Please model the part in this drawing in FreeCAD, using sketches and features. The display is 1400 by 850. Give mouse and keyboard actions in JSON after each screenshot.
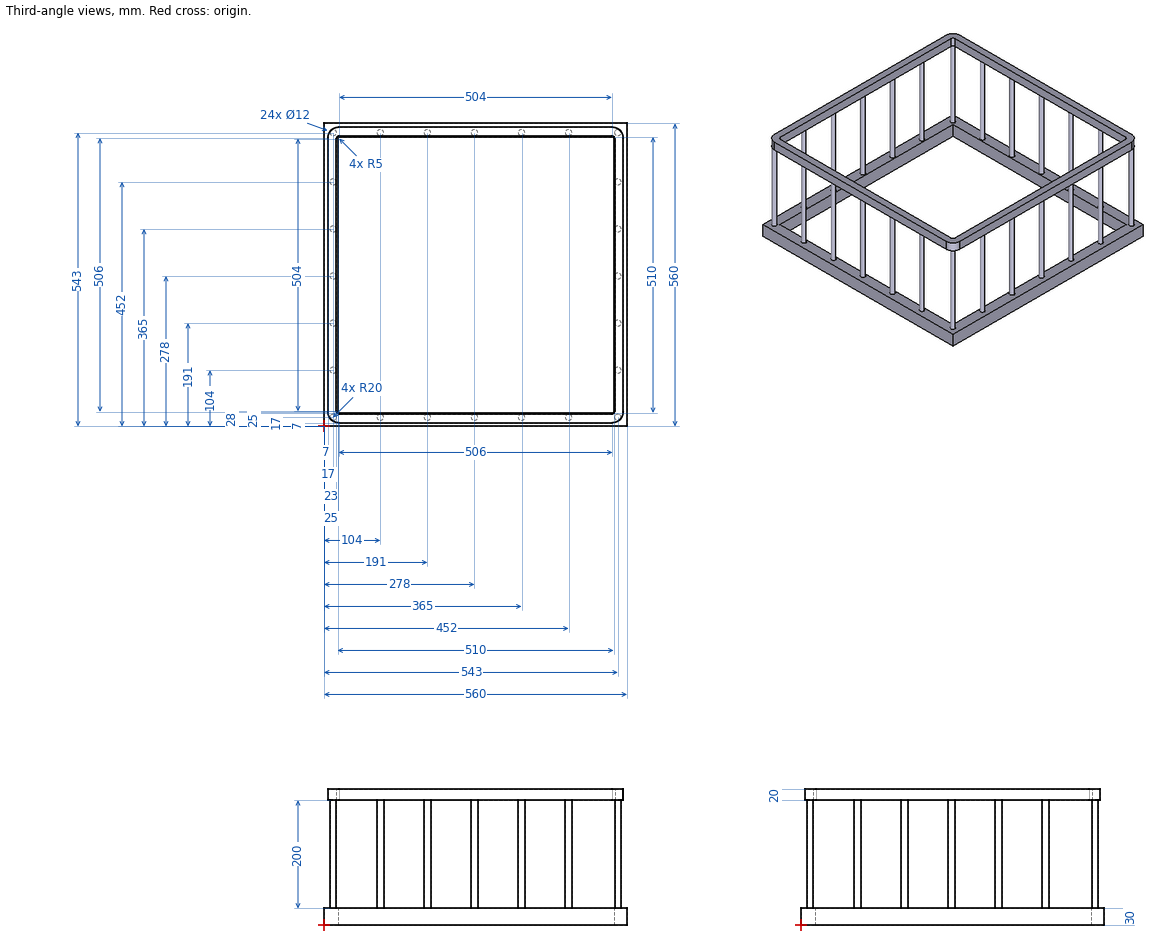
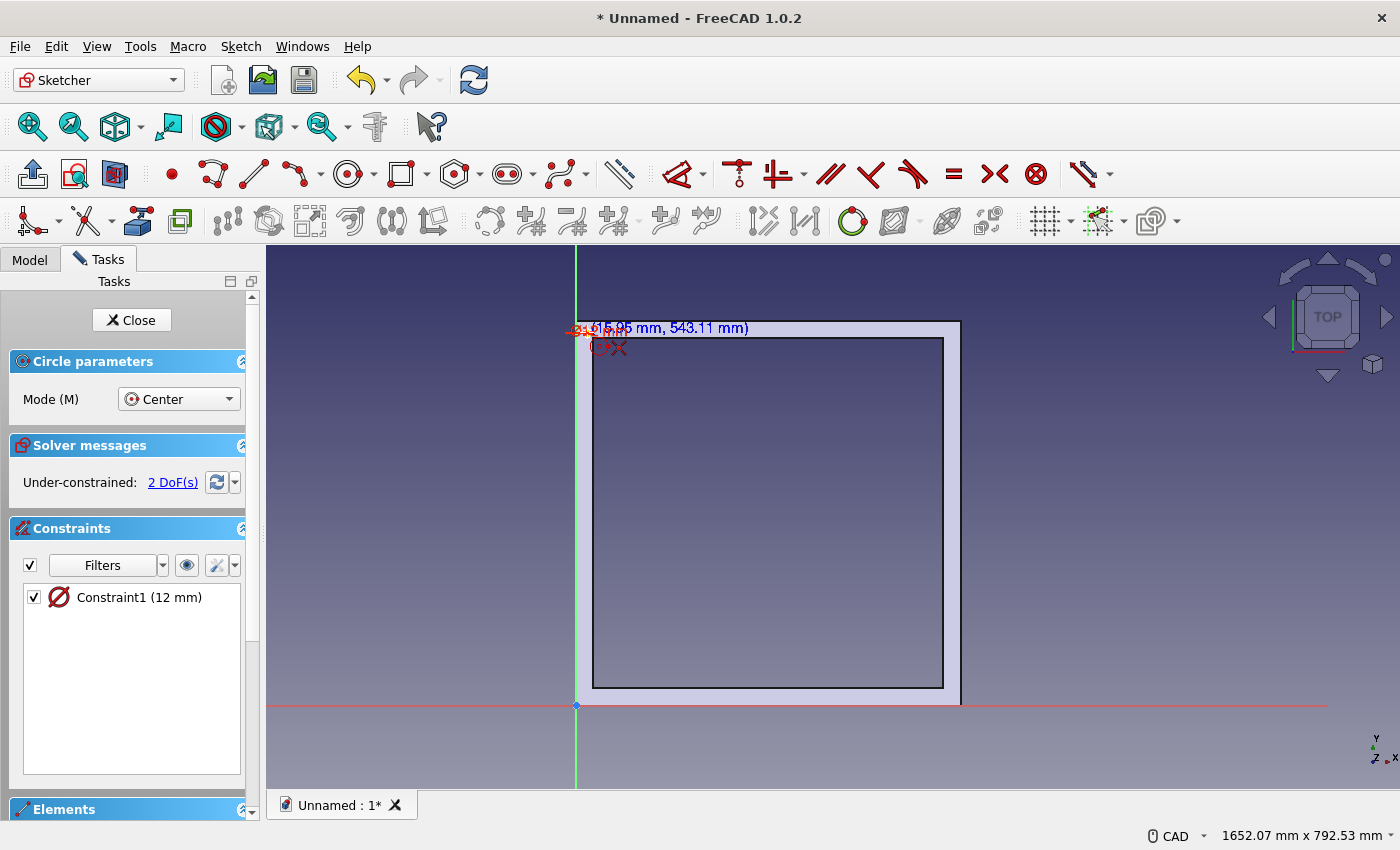
{"action": "scroll", "coordinate": [588, 694], "scroll_direction": "up", "scroll_amount": 9}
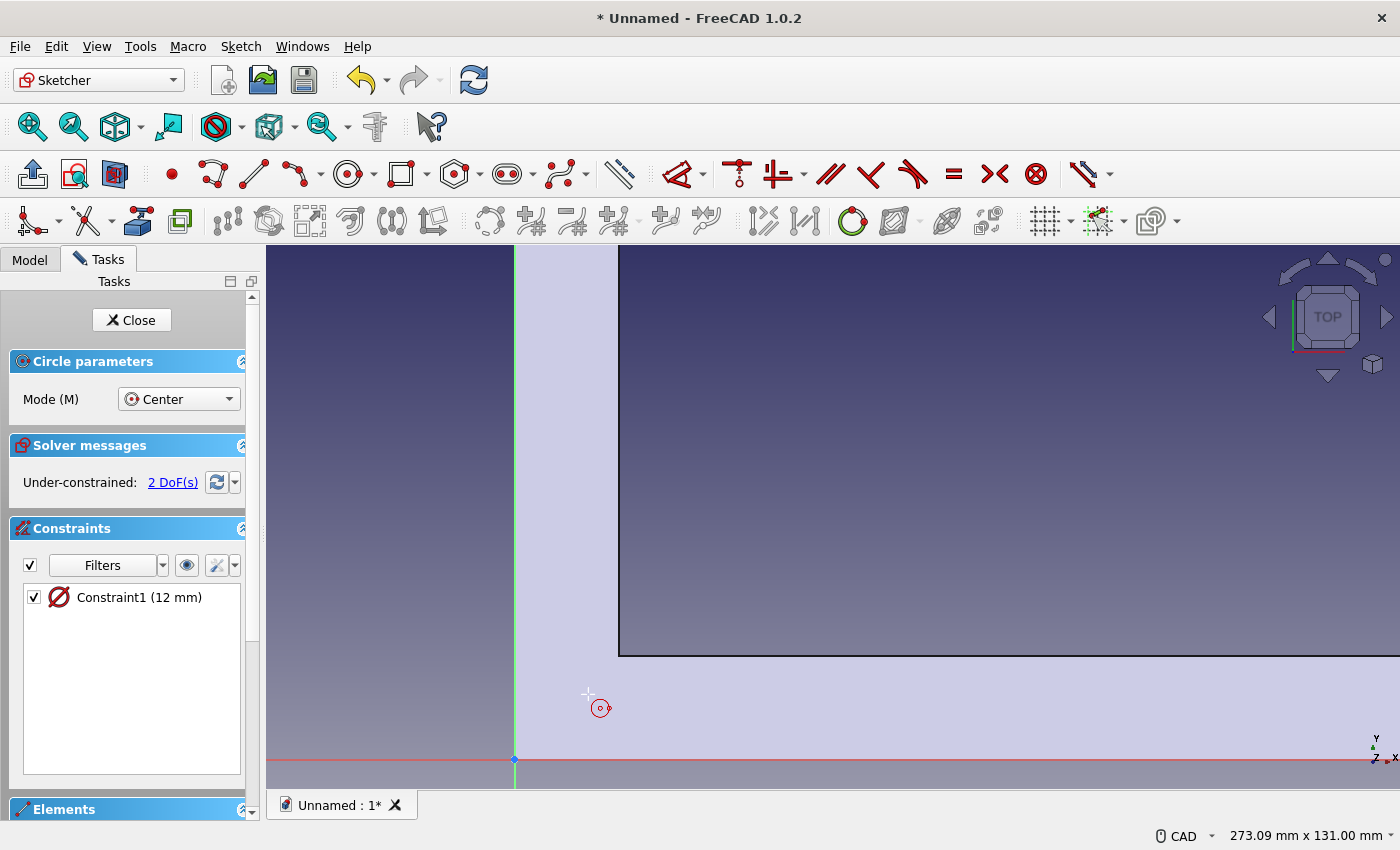
{"action": "scroll", "coordinate": [588, 695], "scroll_direction": "down", "scroll_amount": 9}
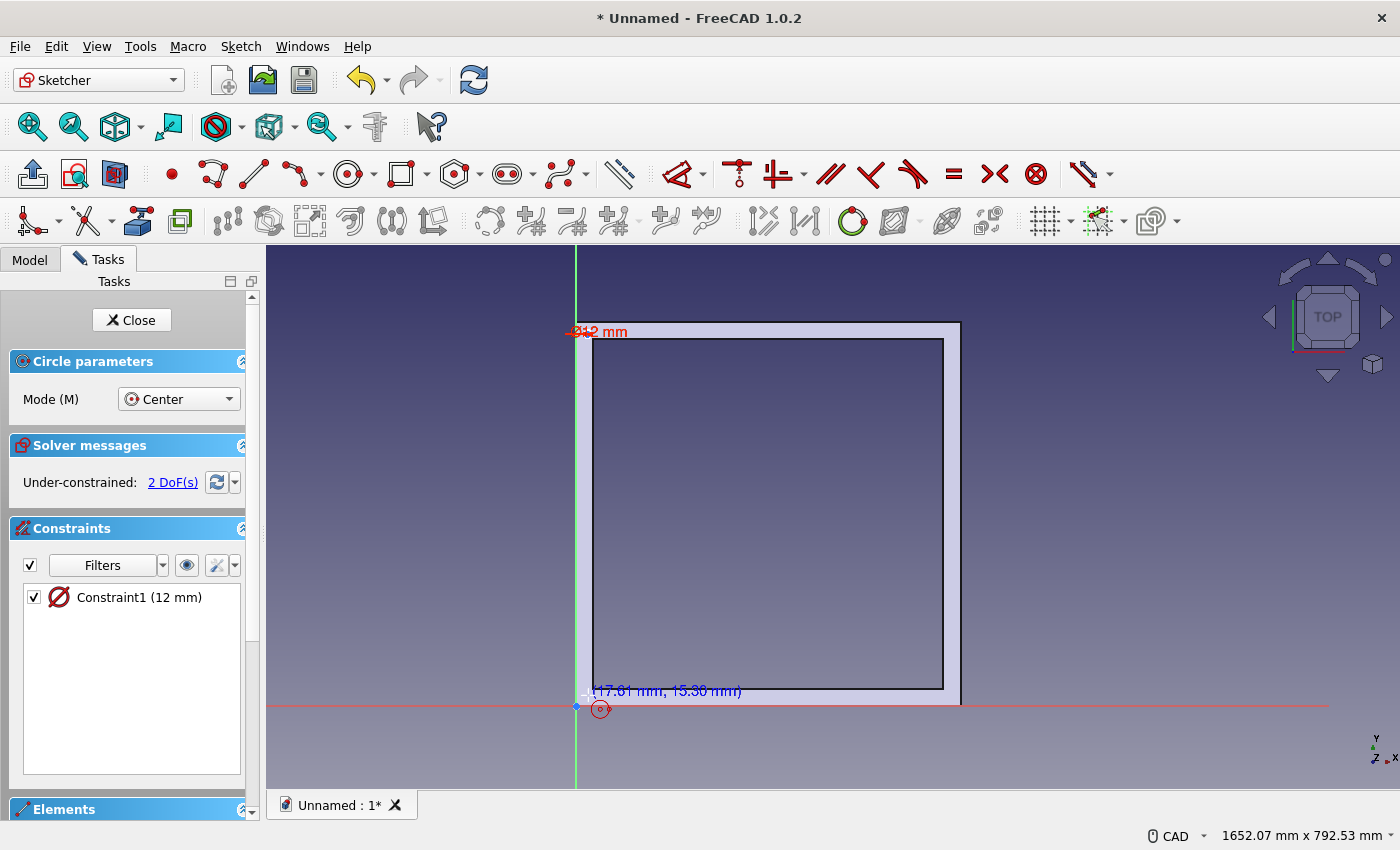
{"action": "scroll", "coordinate": [588, 695], "scroll_direction": "up", "scroll_amount": 2}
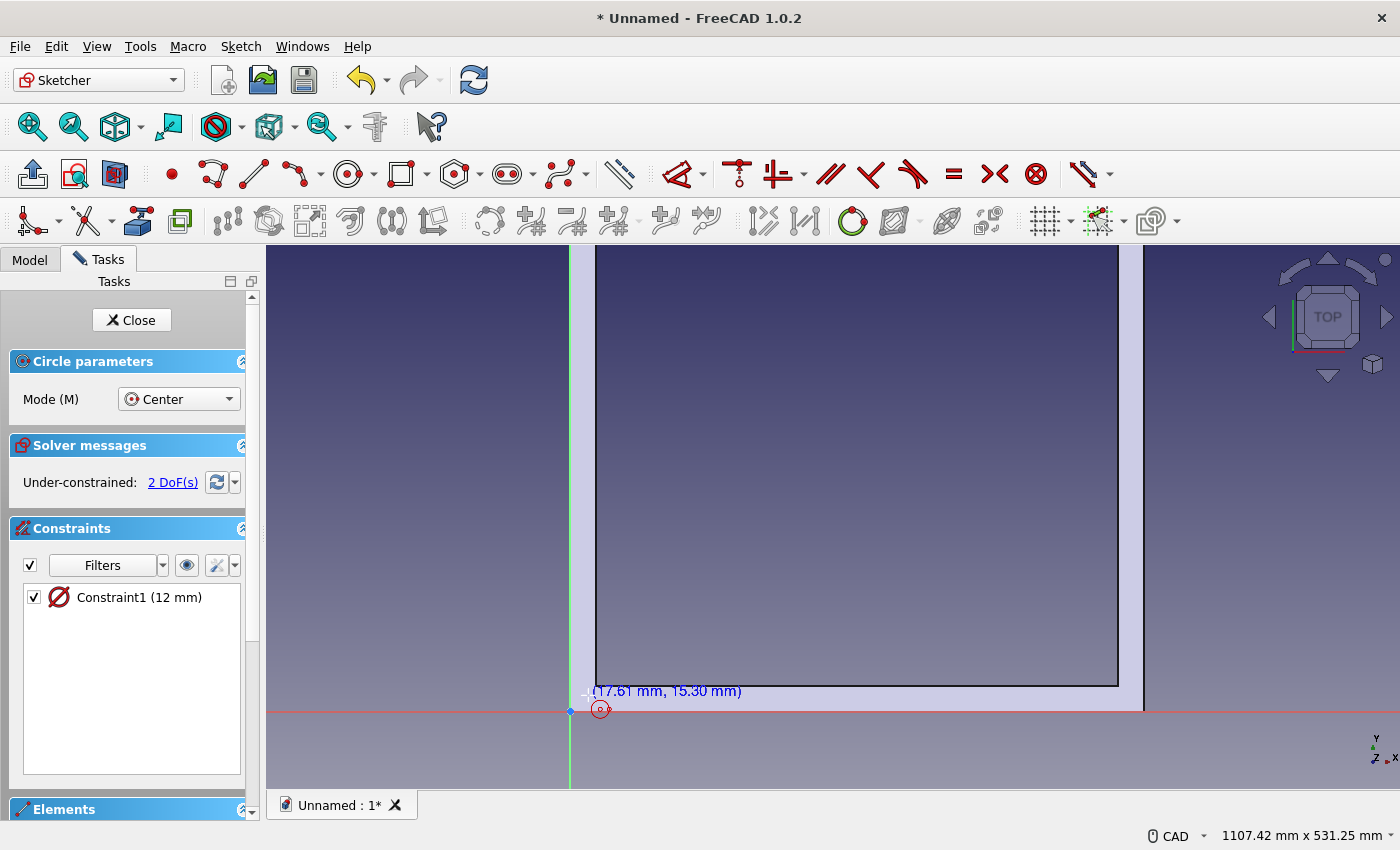
{"action": "left_click", "coordinate": [588, 694]}
{"action": "mouse_move", "coordinate": [592, 690]}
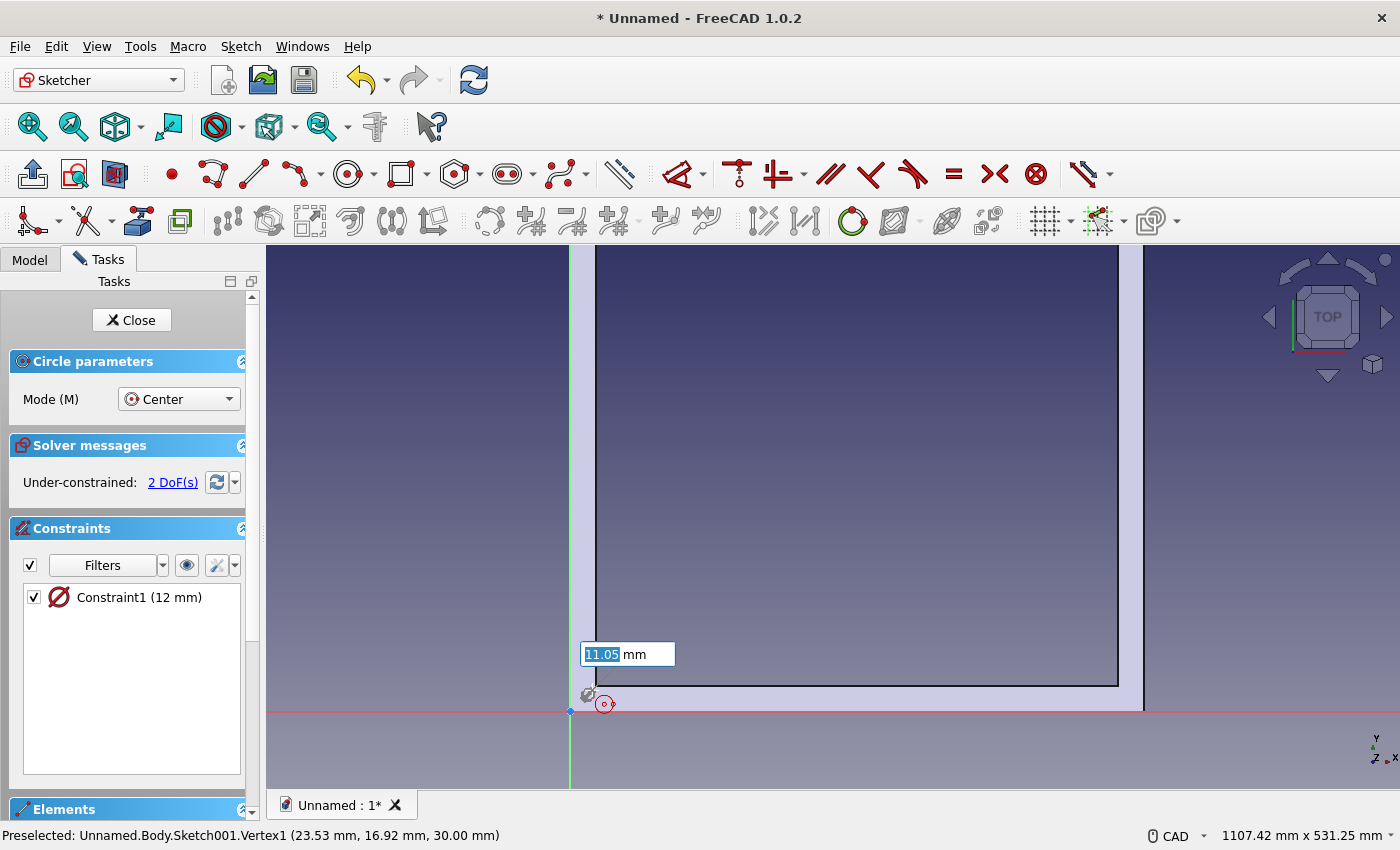
{"action": "type", "text": "12"}
{"action": "key", "text": "Return"}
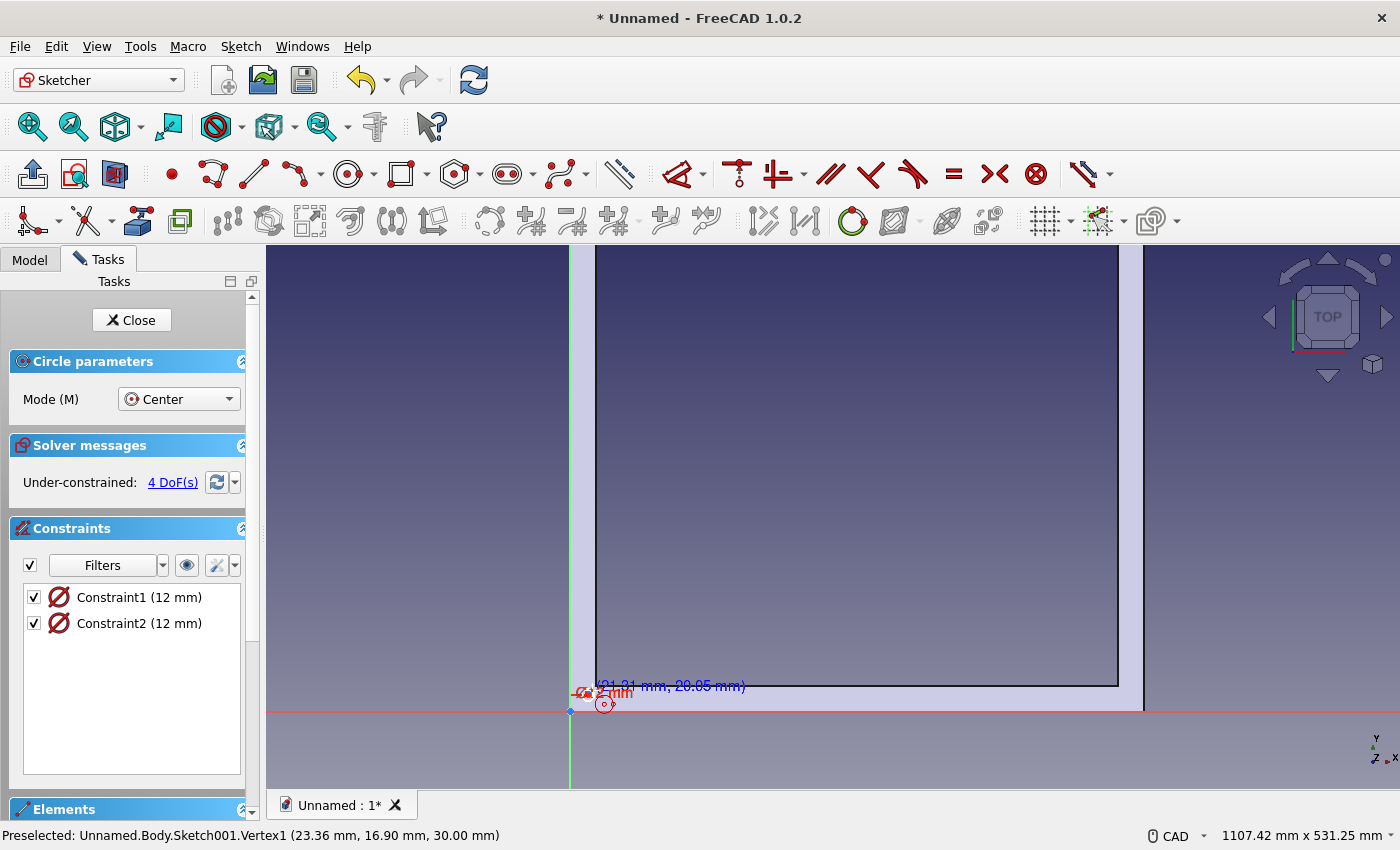
{"action": "scroll", "coordinate": [1126, 694], "scroll_direction": "up", "scroll_amount": 7}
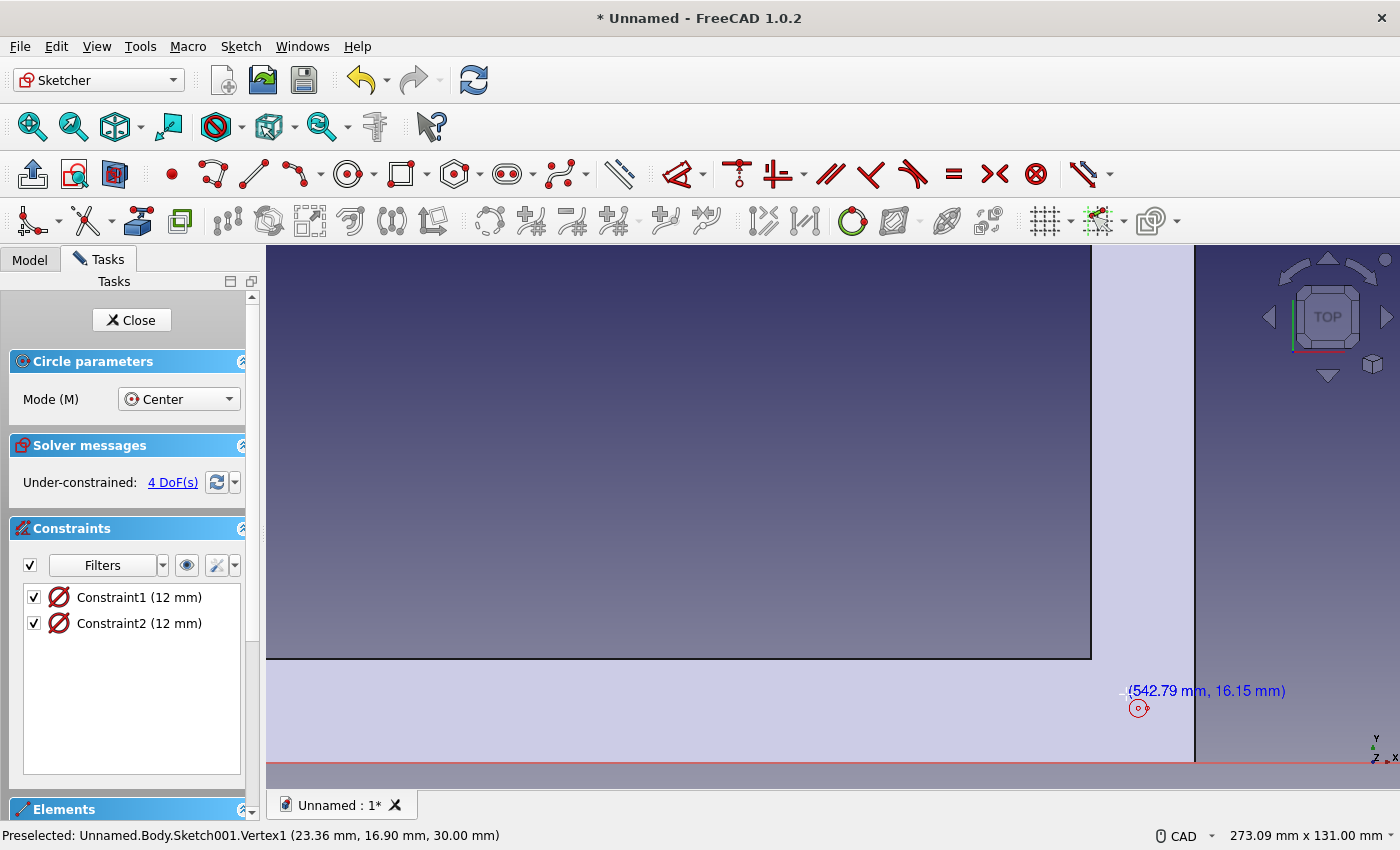
{"action": "scroll", "coordinate": [914, 694], "scroll_direction": "down", "scroll_amount": 9}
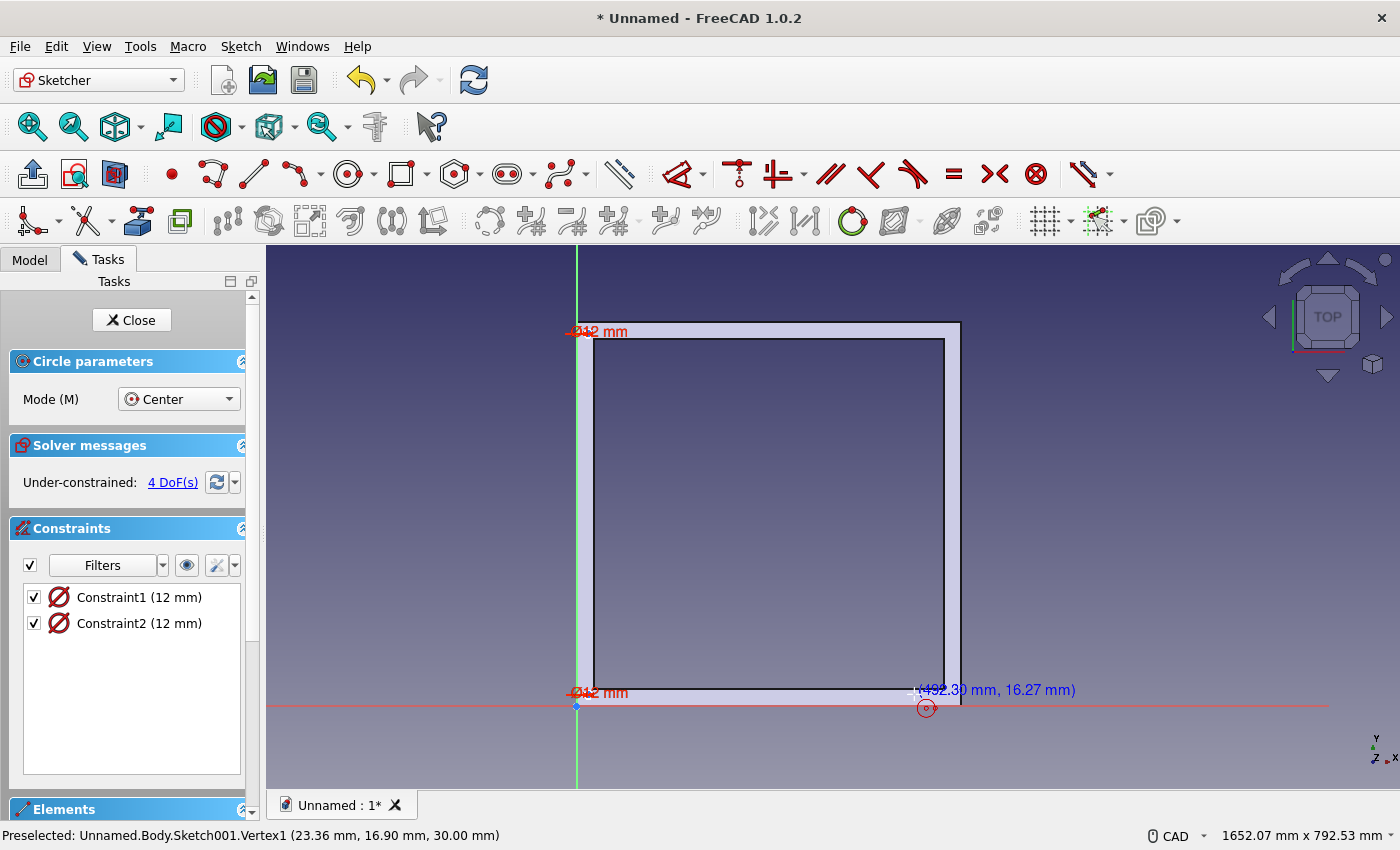
{"action": "scroll", "coordinate": [949, 694], "scroll_direction": "up", "scroll_amount": 2}